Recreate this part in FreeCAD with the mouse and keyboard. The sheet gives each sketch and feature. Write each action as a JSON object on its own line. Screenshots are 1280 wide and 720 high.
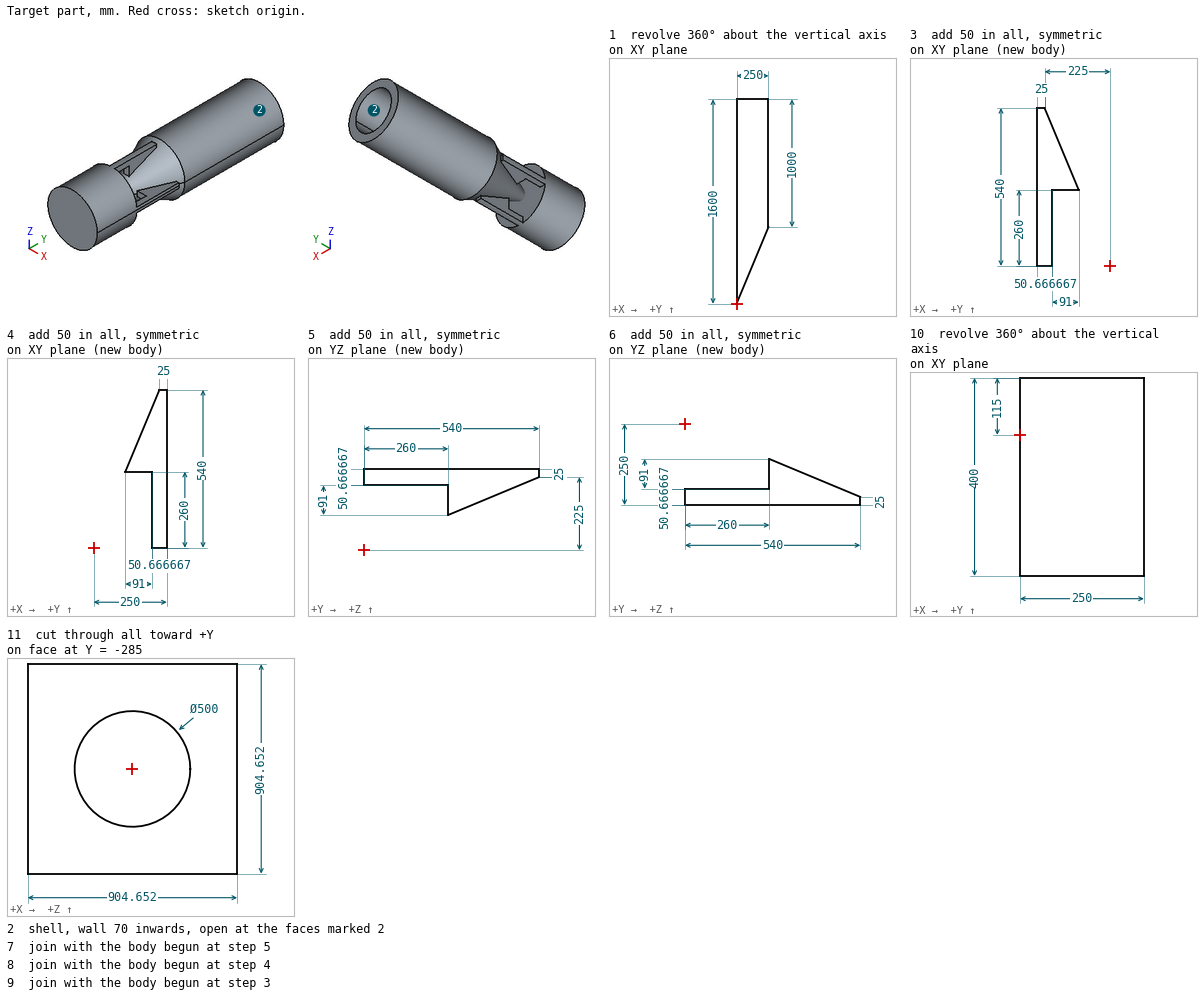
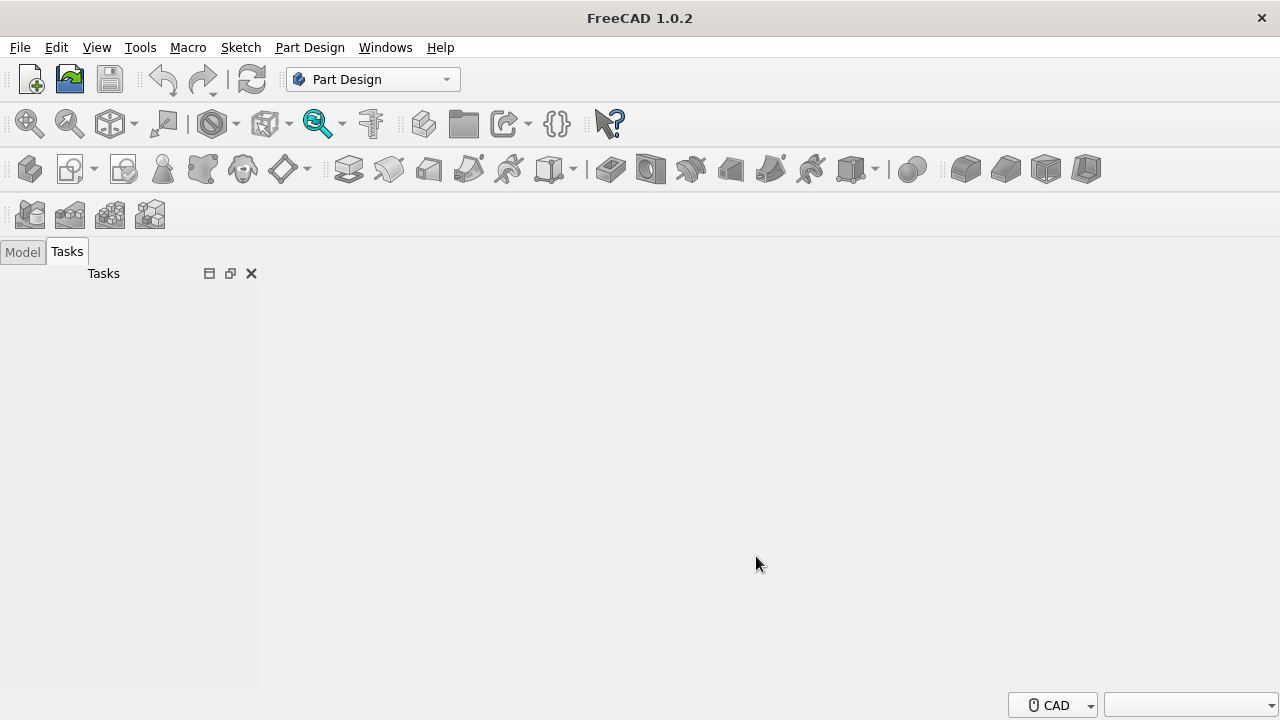
{"action": "left_click", "coordinate": [30, 80]}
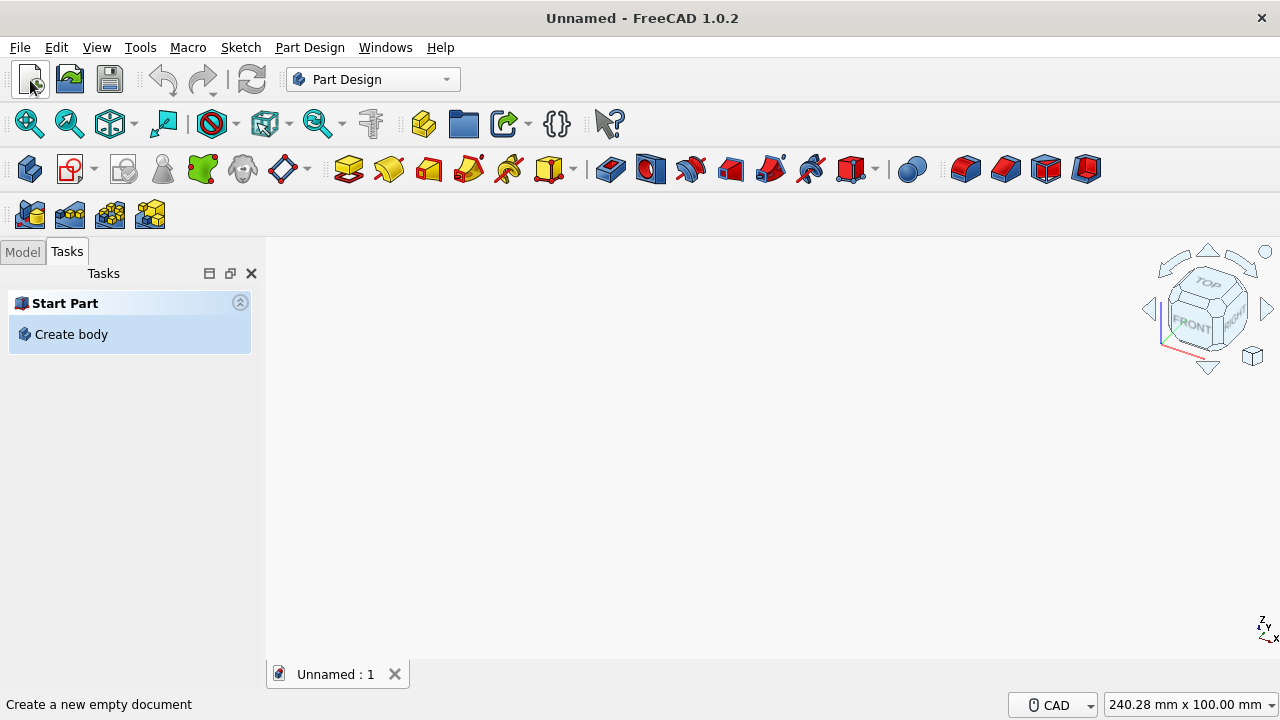
{"action": "left_click", "coordinate": [70, 170]}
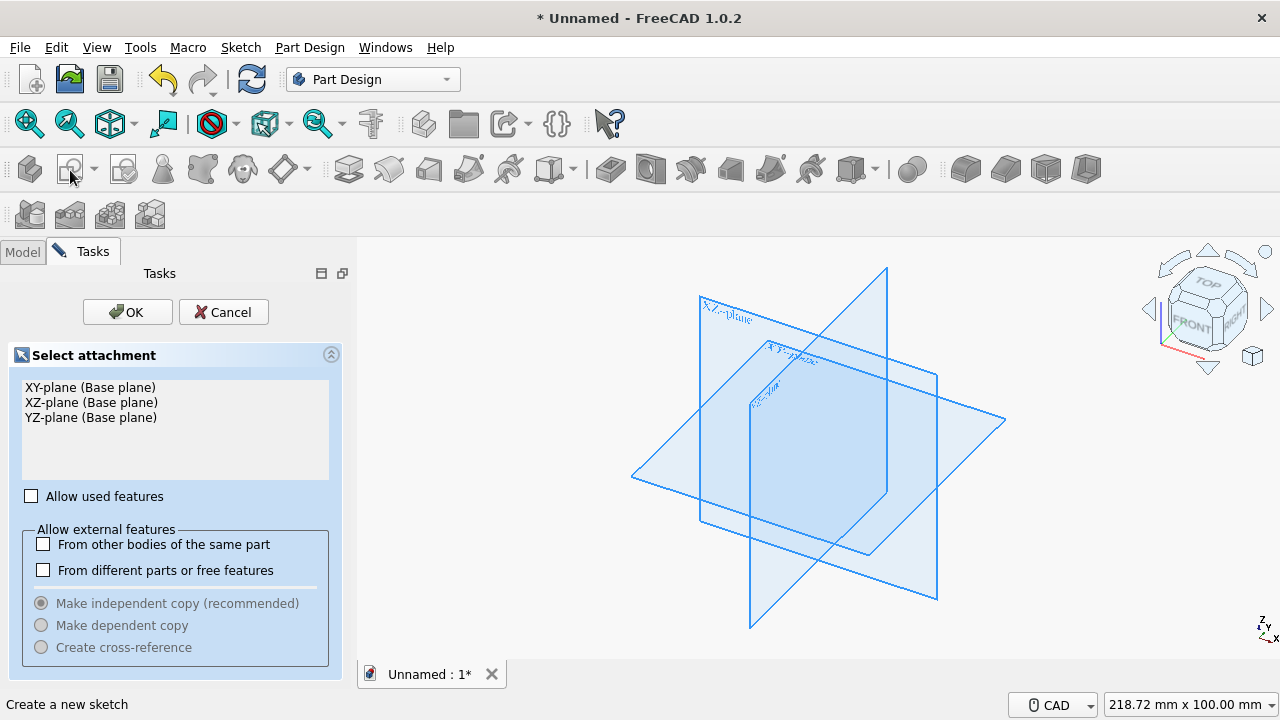
{"action": "left_click", "coordinate": [82, 388]}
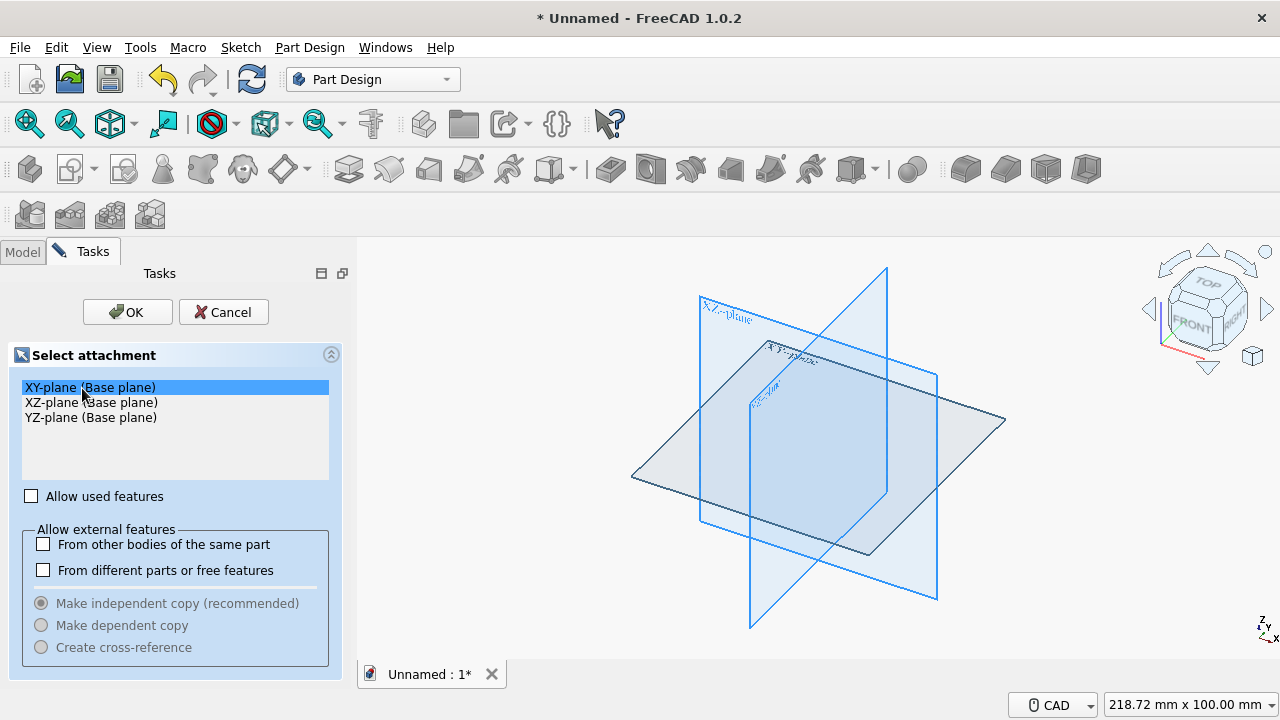
{"action": "left_click", "coordinate": [128, 312]}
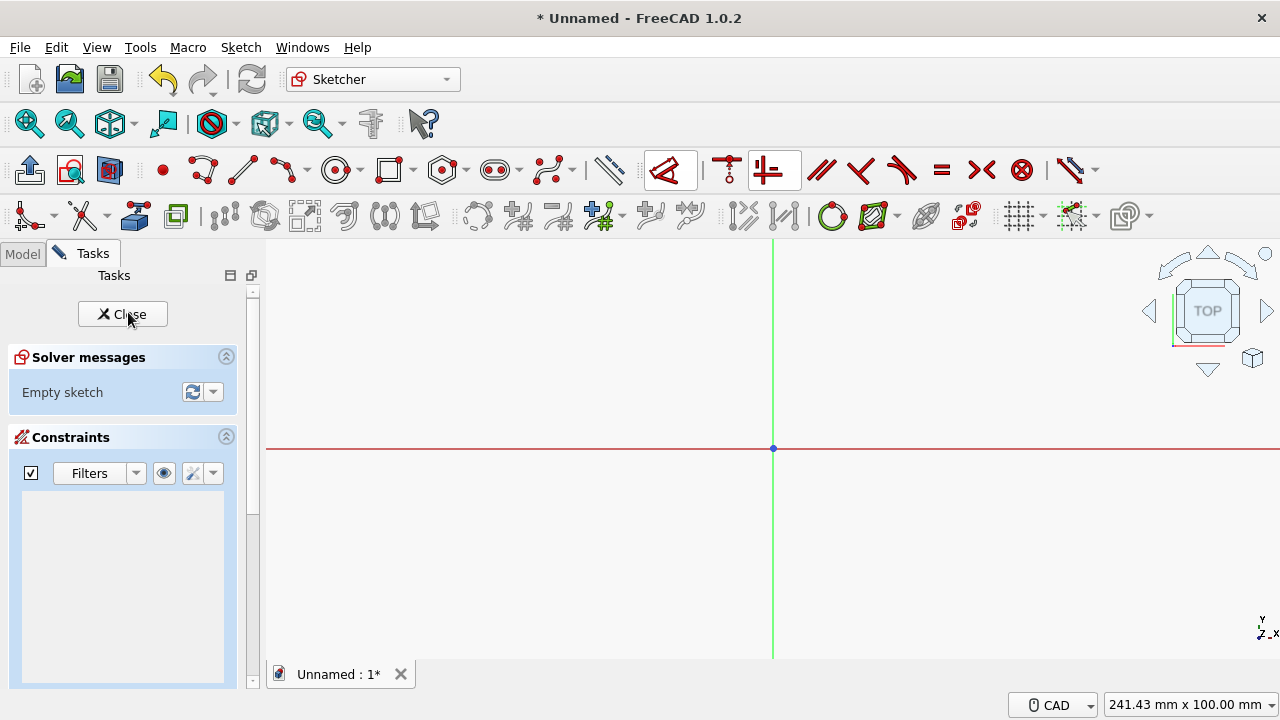
{"action": "scroll", "coordinate": [679, 592], "scroll_direction": "down", "scroll_amount": 16}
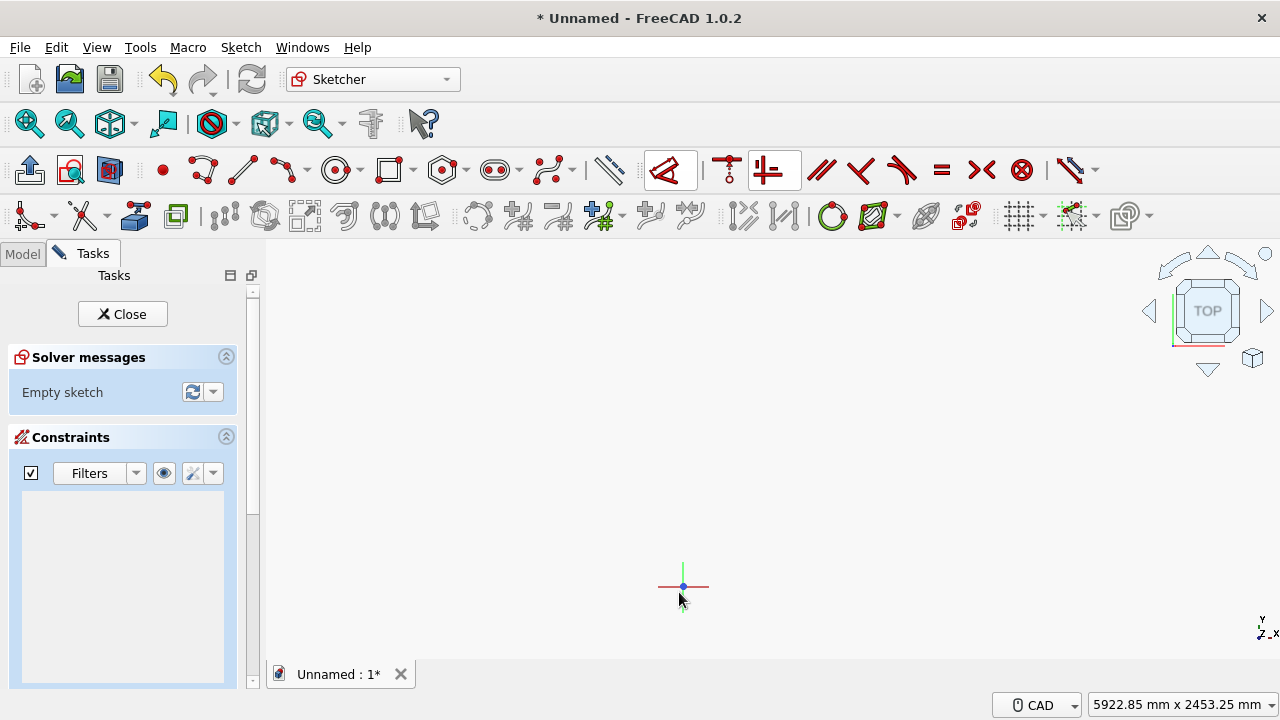
{"action": "left_click", "coordinate": [204, 170]}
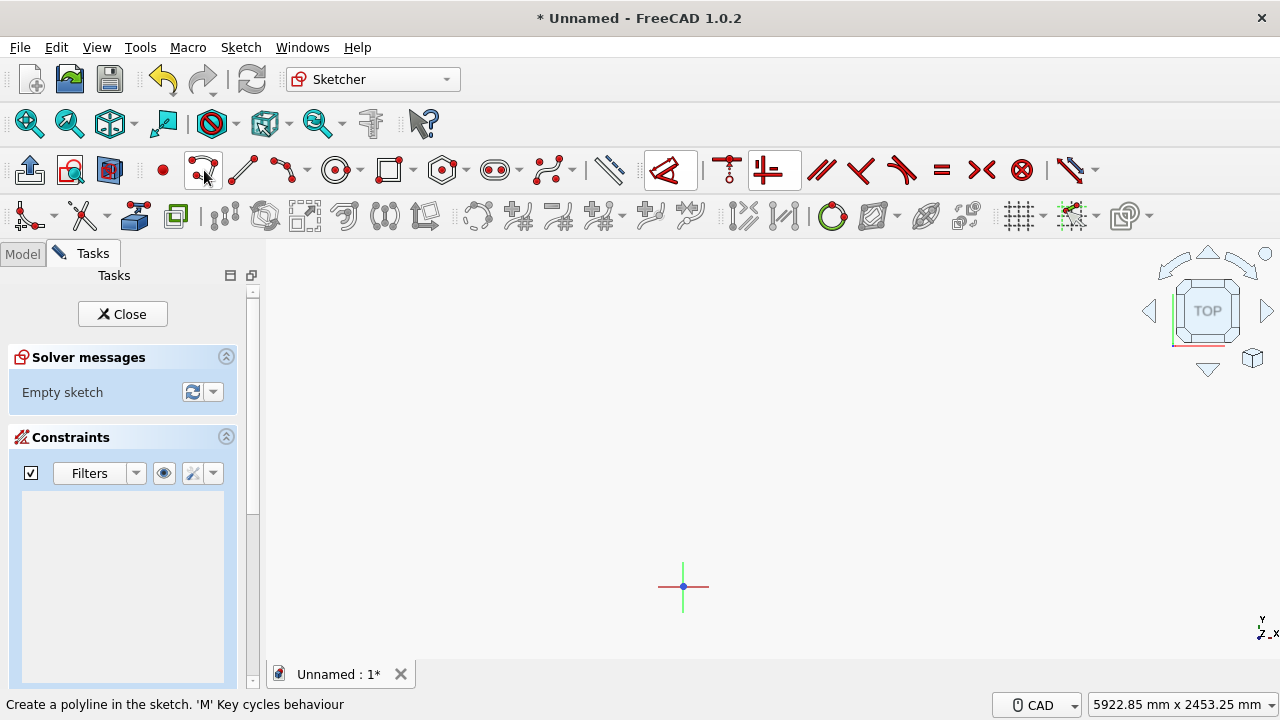
{"action": "left_click", "coordinate": [683, 587]}
{"action": "left_click", "coordinate": [726, 484]}
{"action": "left_click", "coordinate": [726, 313]}
{"action": "left_click", "coordinate": [692, 313]}
{"action": "left_click", "coordinate": [683, 587]}
{"action": "key", "text": "Escape"}
{"action": "key", "text": "Escape"}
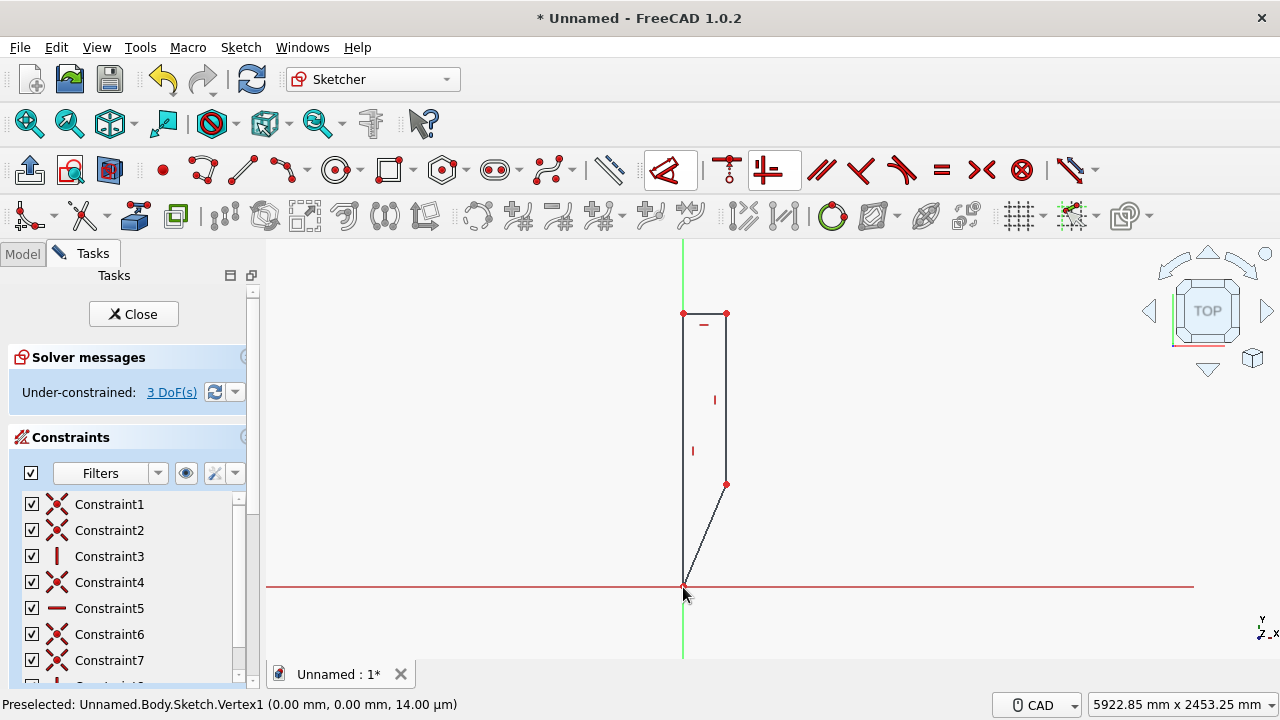
{"action": "left_click", "coordinate": [664, 170]}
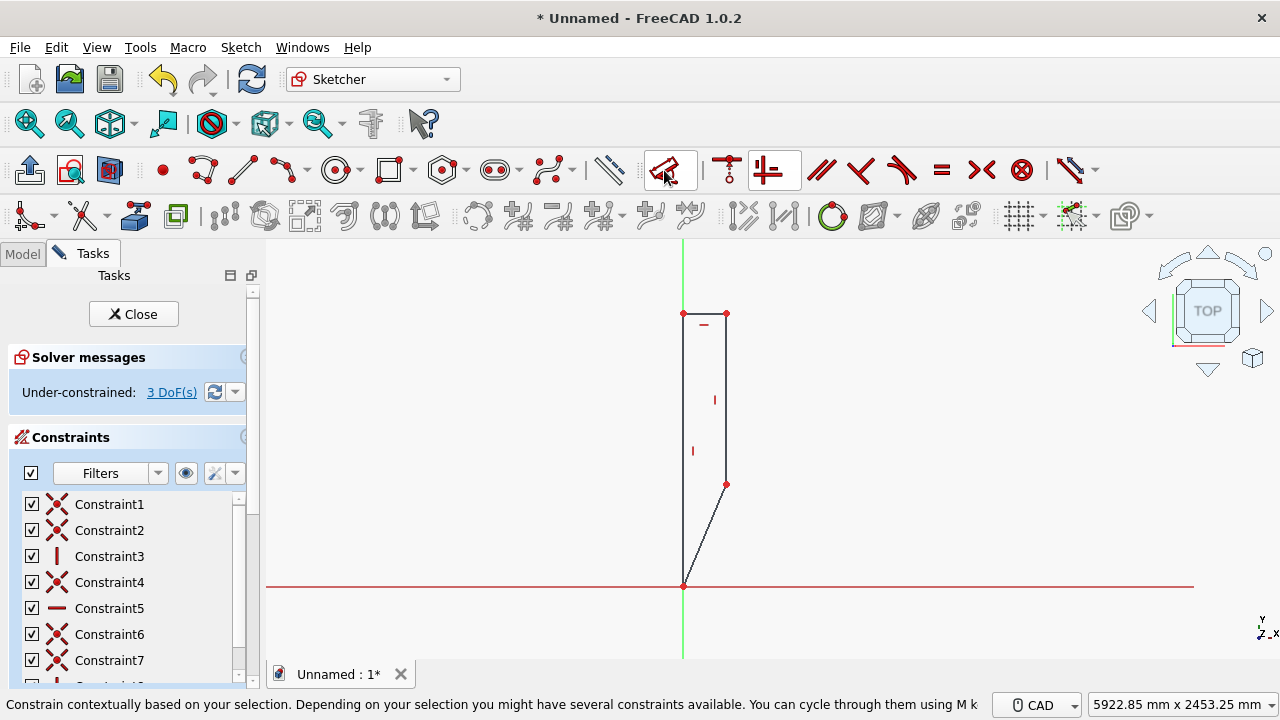
{"action": "left_click", "coordinate": [713, 314]}
{"action": "left_click", "coordinate": [705, 280]}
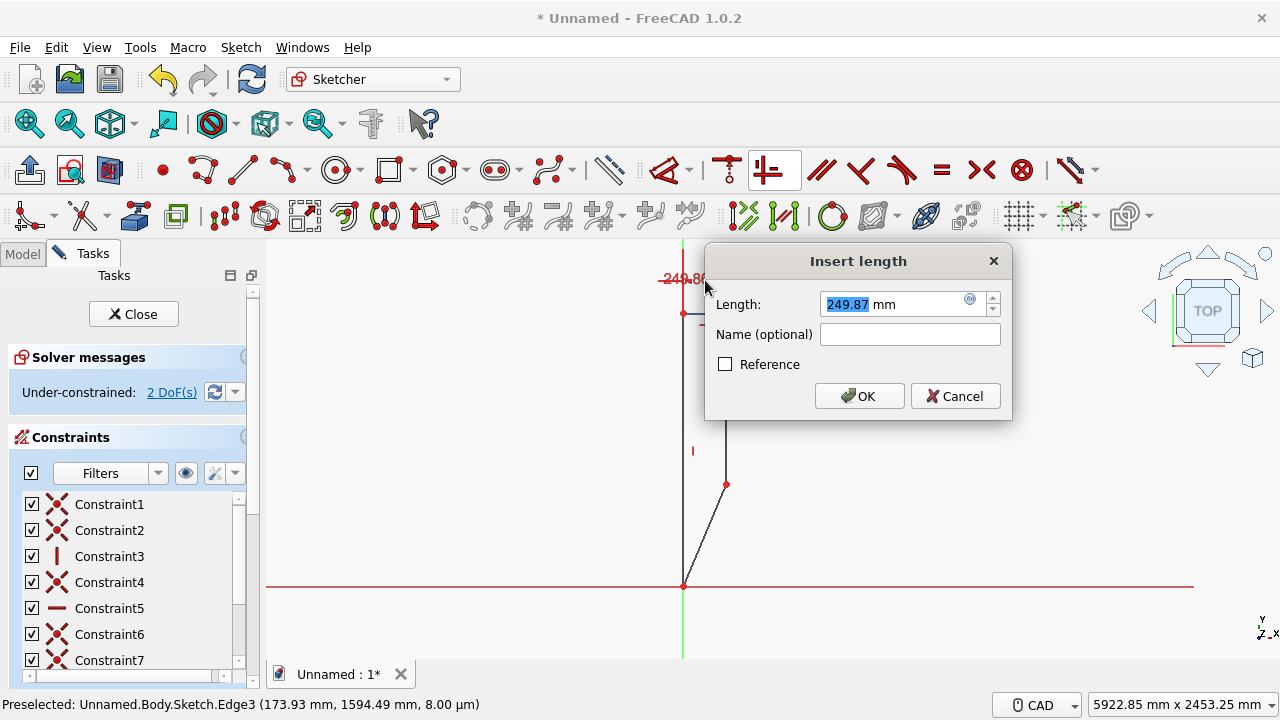
{"action": "type", "text": "250"}
{"action": "key", "text": "Return"}